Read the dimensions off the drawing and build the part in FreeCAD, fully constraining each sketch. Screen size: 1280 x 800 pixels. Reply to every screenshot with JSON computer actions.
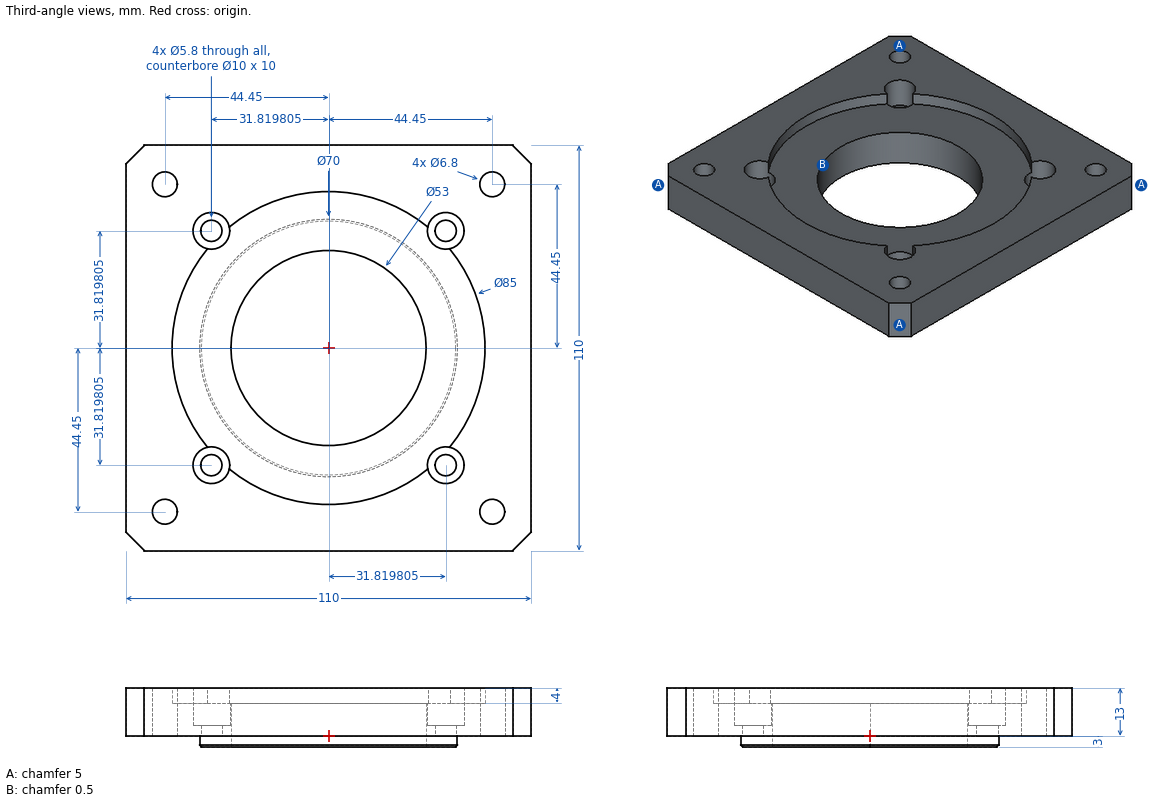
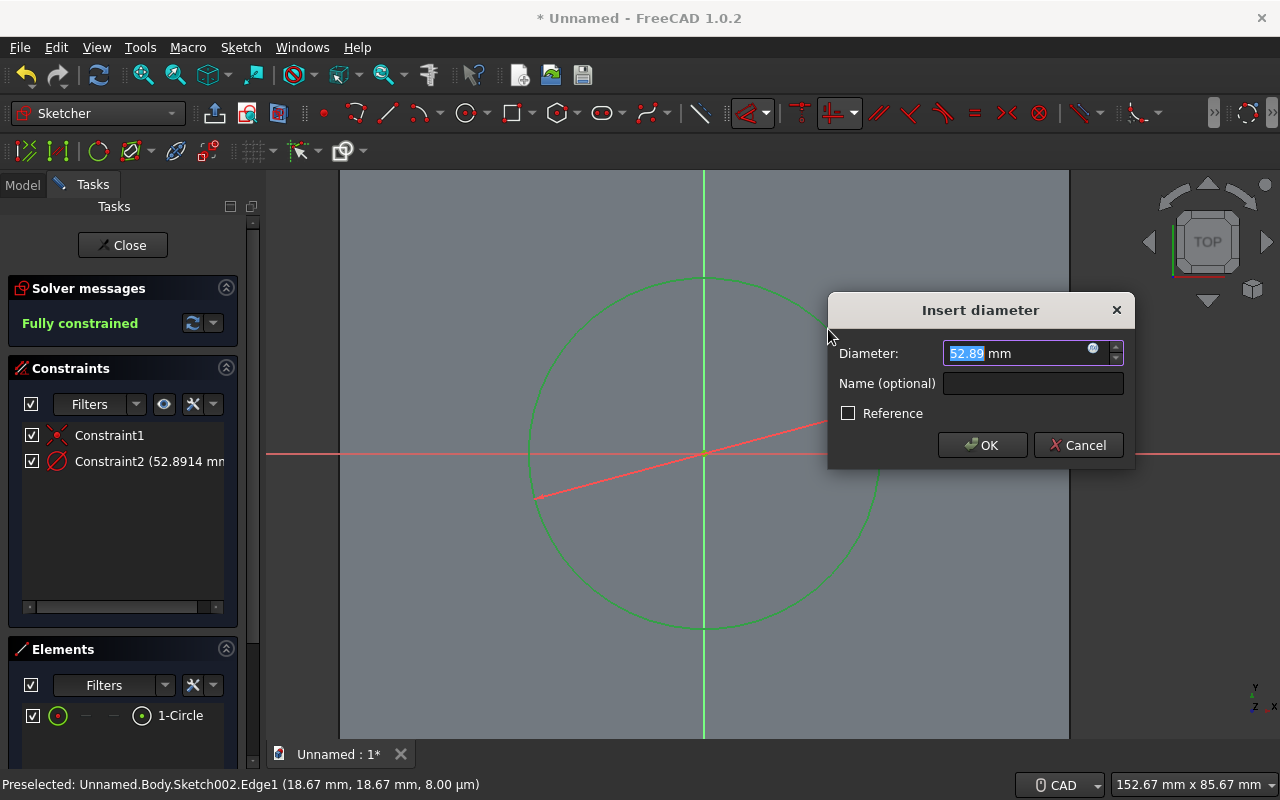
{"action": "type", "text": "53"}
{"action": "key", "text": "Return"}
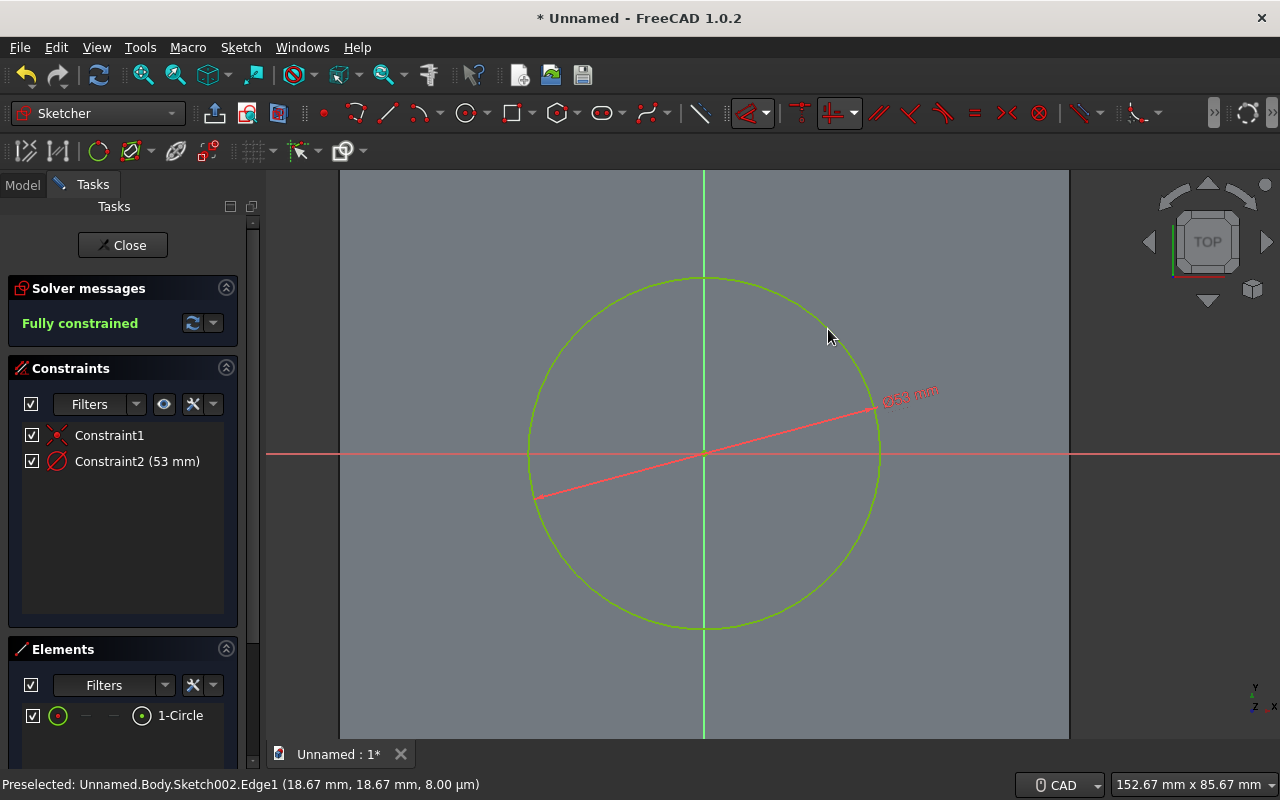
{"action": "left_click", "coordinate": [123, 245]}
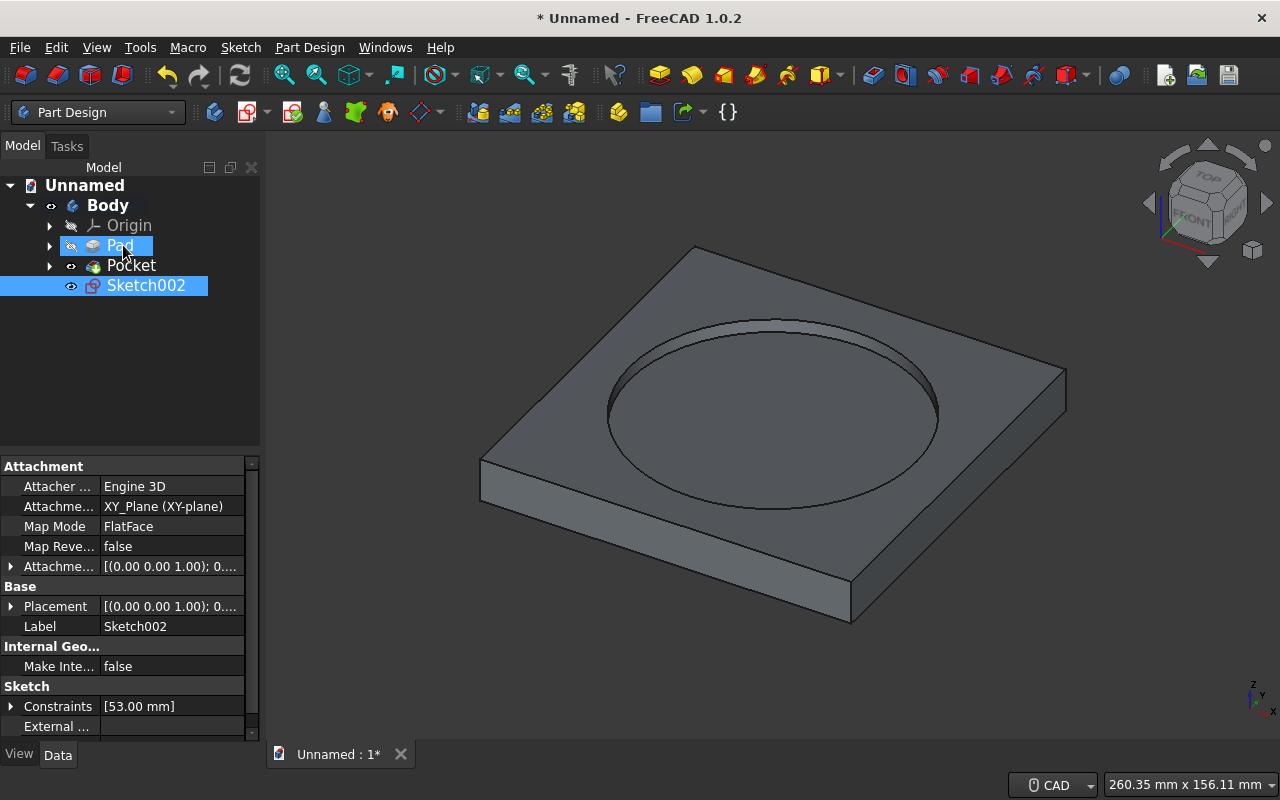
{"action": "left_click", "coordinate": [874, 76]}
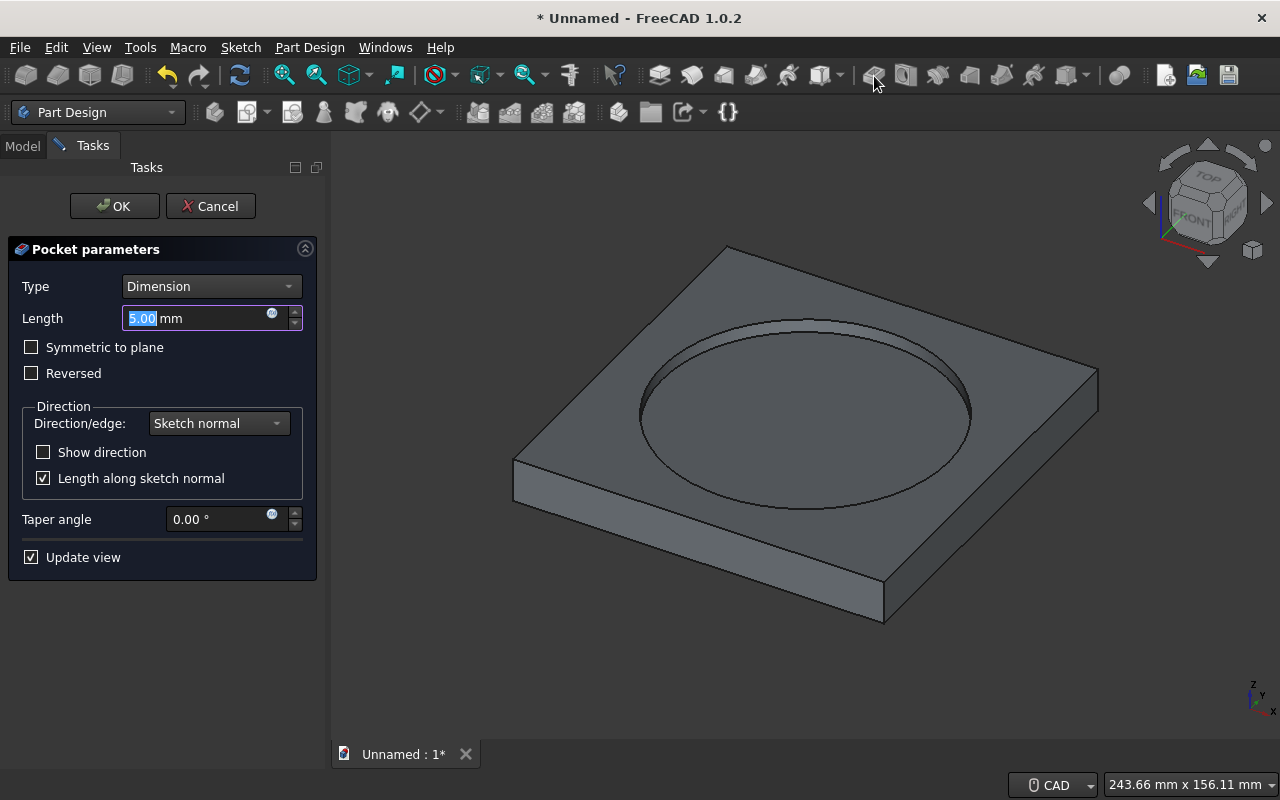
{"action": "left_click", "coordinate": [212, 286]}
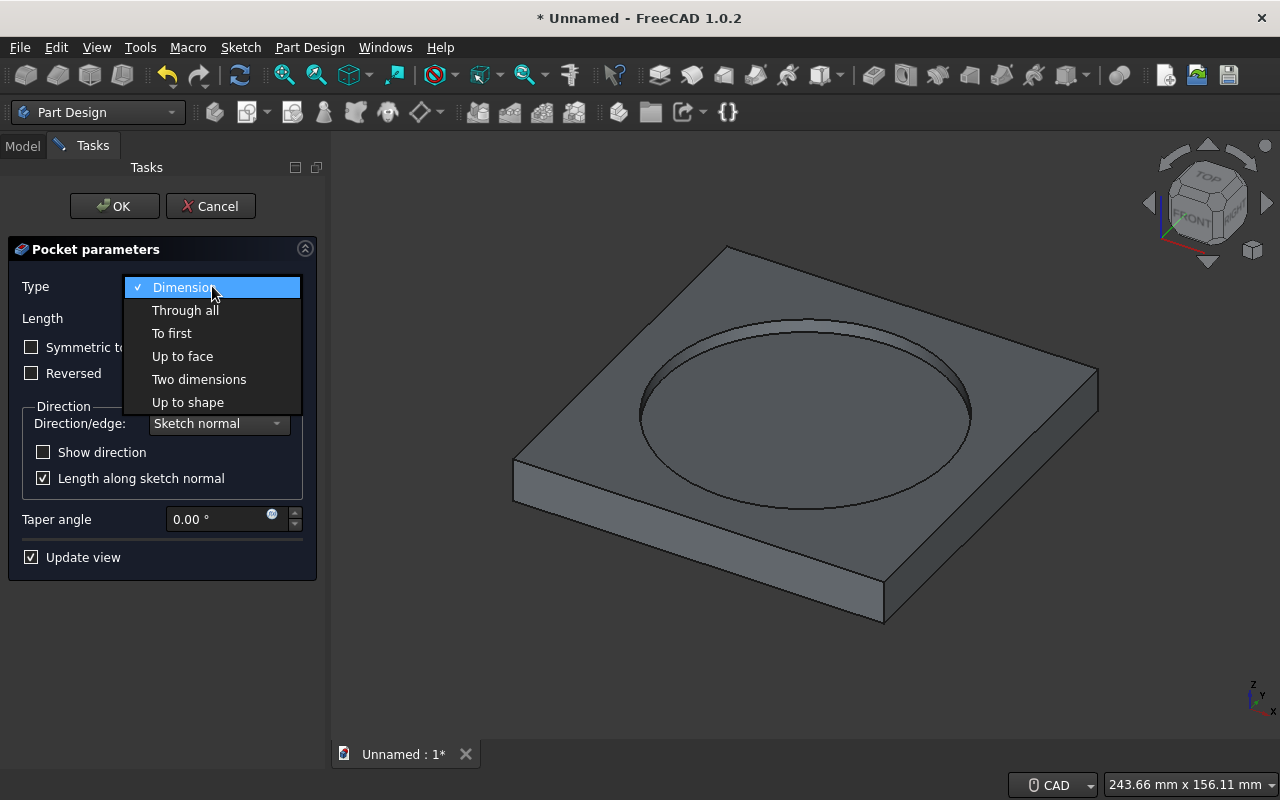
{"action": "left_click", "coordinate": [212, 310]}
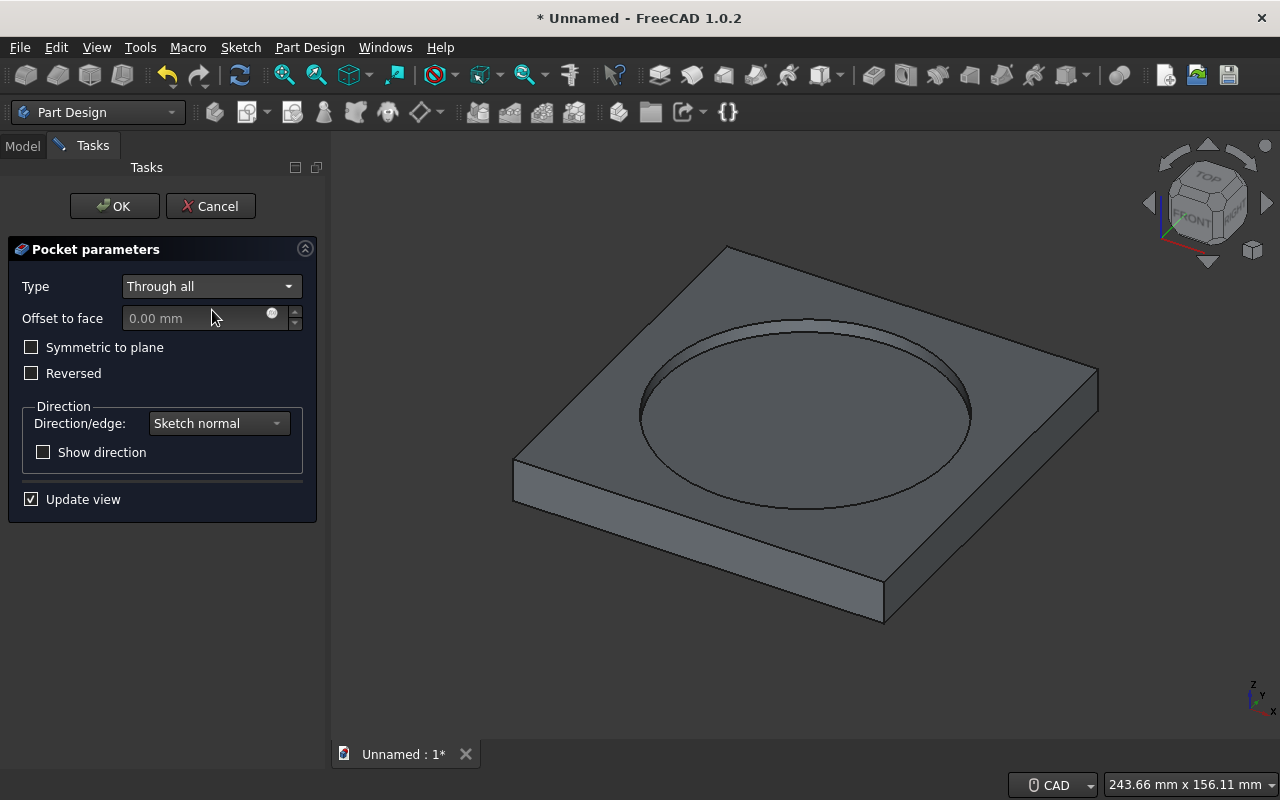
{"action": "left_click", "coordinate": [30, 373]}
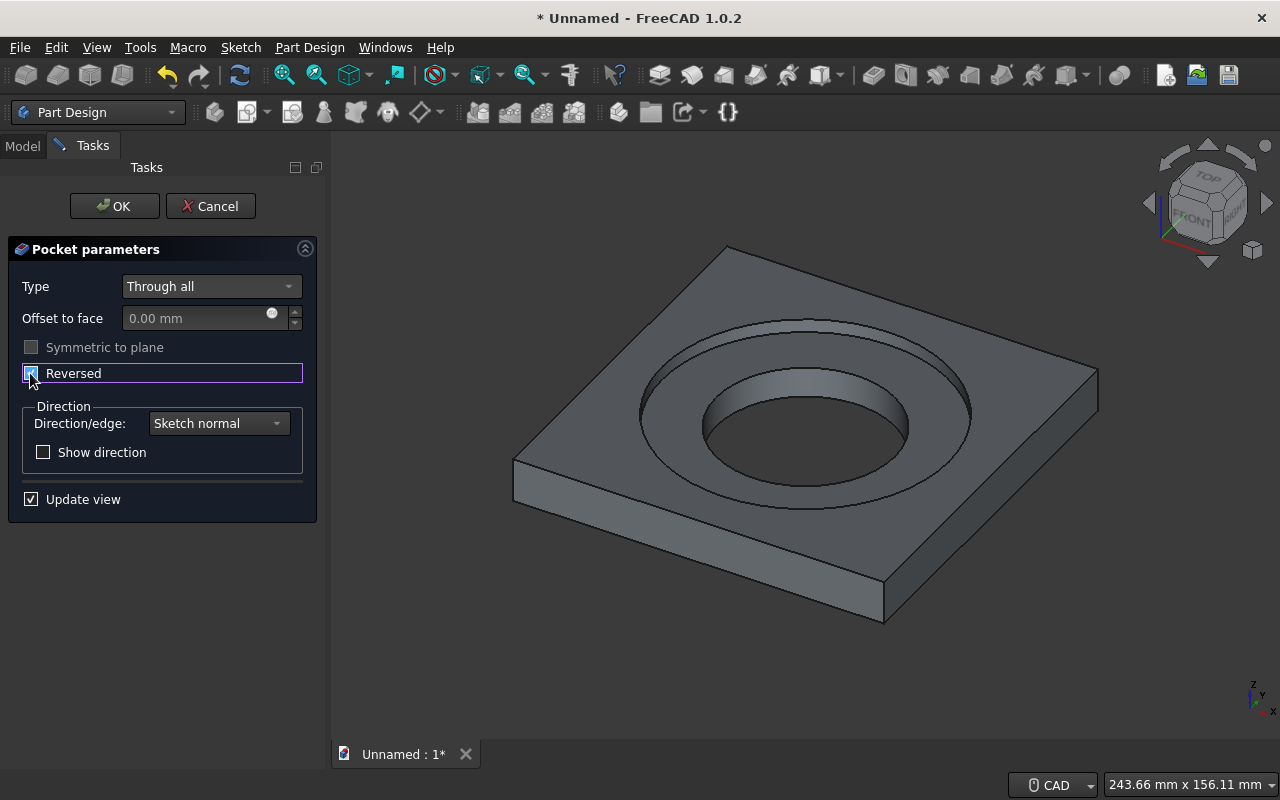
{"action": "left_click", "coordinate": [115, 206]}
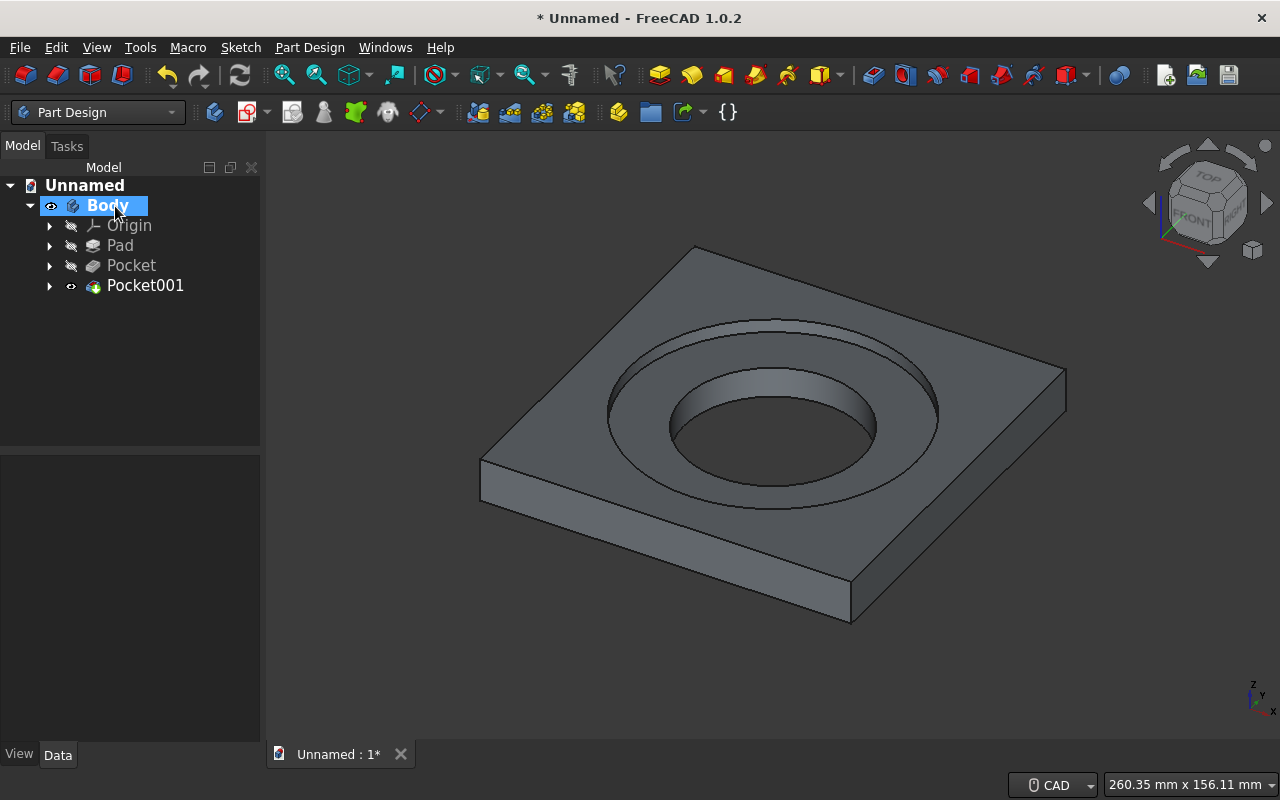
{"action": "left_click", "coordinate": [50, 226]}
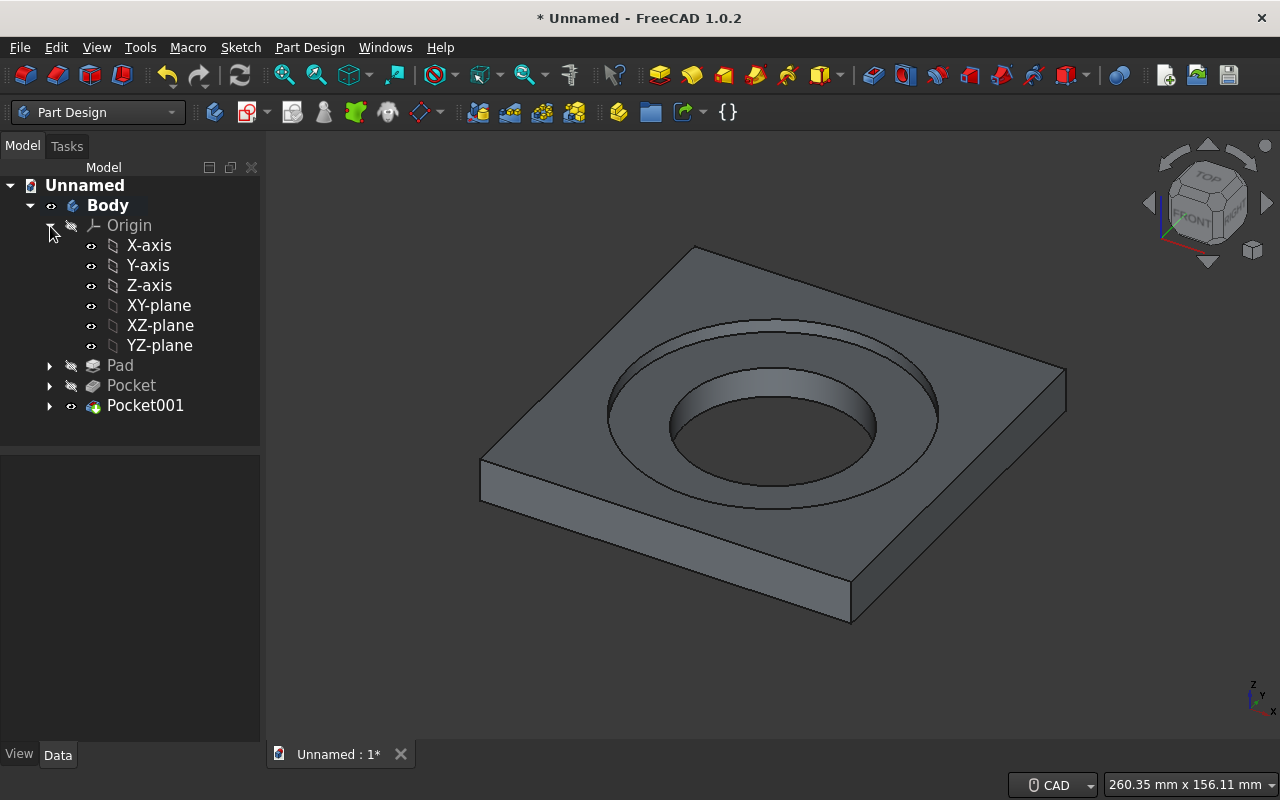
{"action": "left_click", "coordinate": [136, 306]}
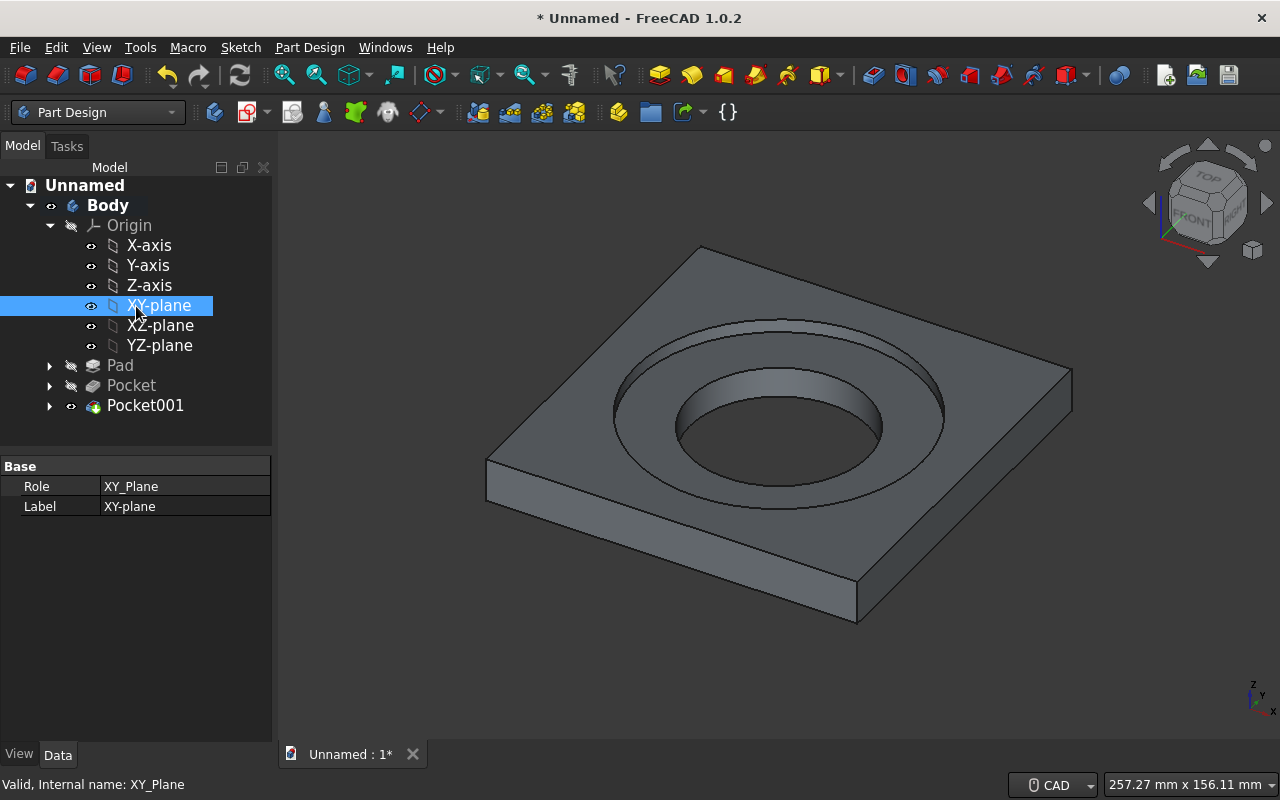
{"action": "left_click", "coordinate": [420, 112]}